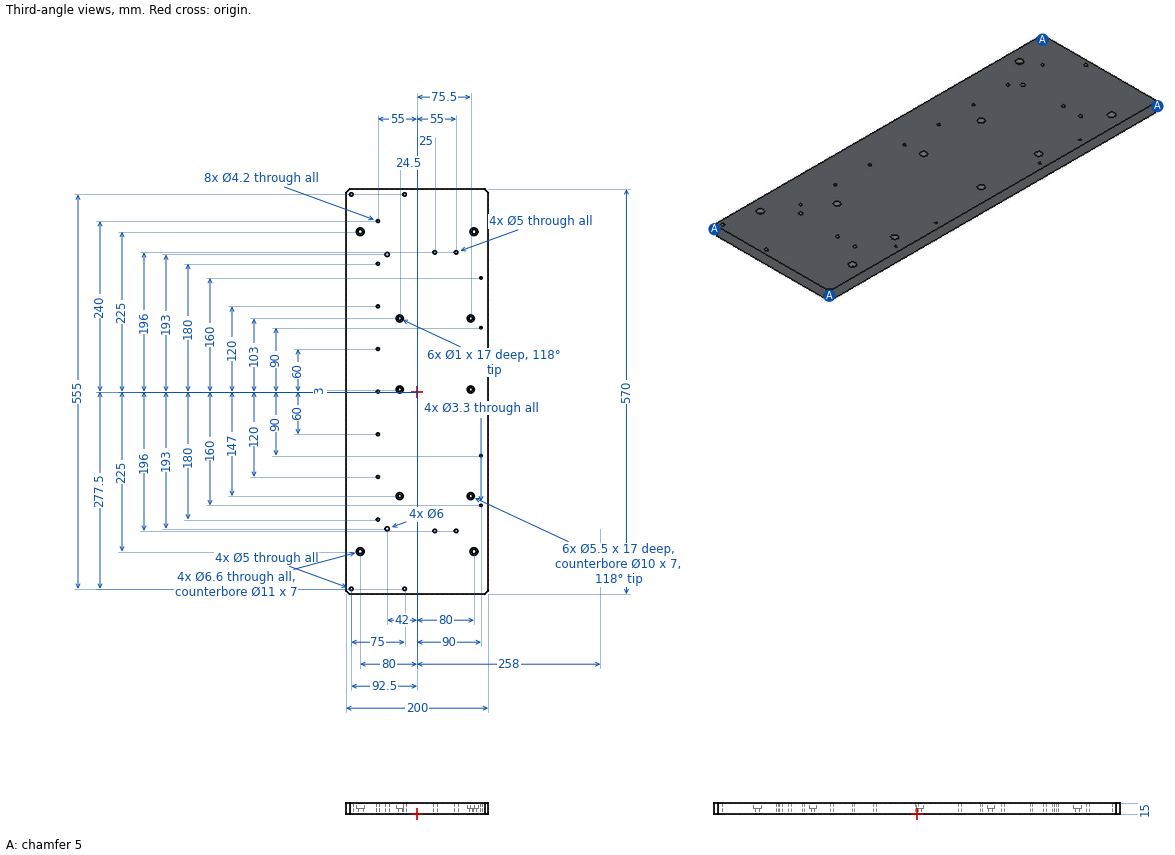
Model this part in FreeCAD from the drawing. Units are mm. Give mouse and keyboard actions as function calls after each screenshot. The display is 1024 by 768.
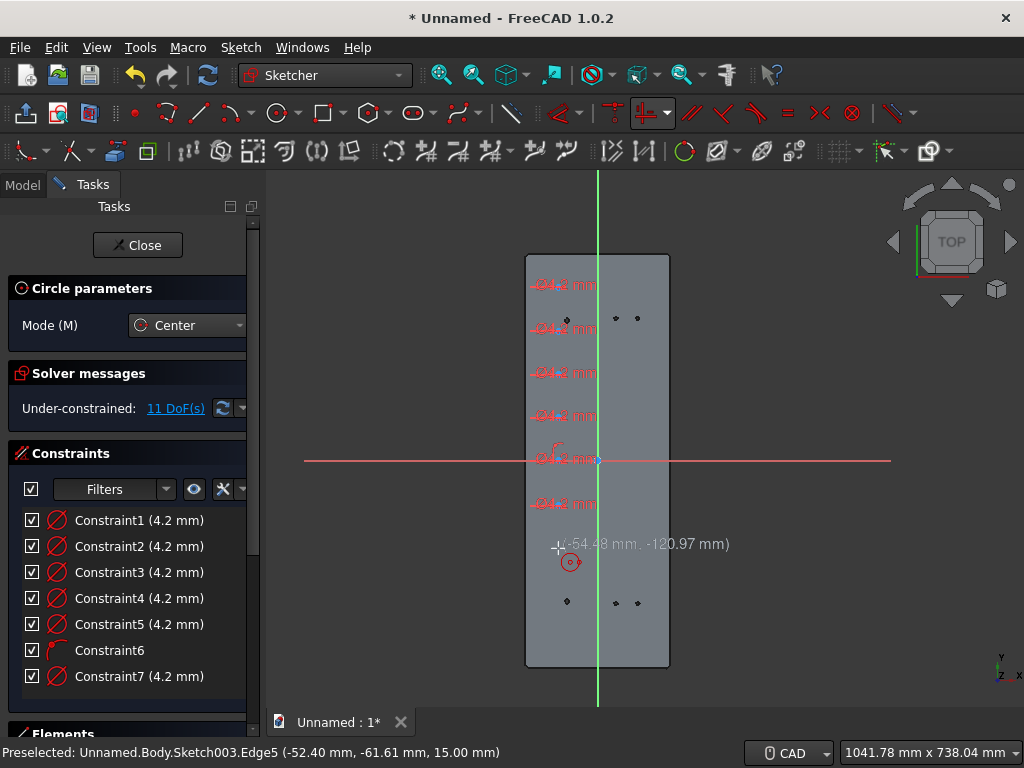
click(558, 548)
move(559, 547)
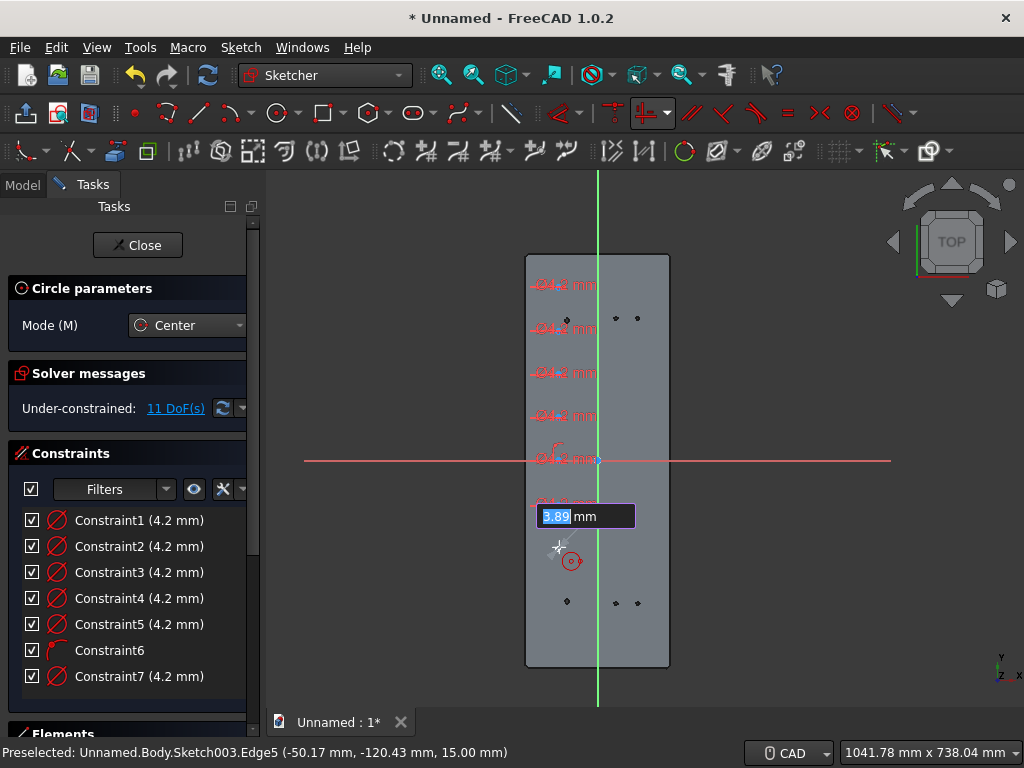
text(4.2)
key(Return)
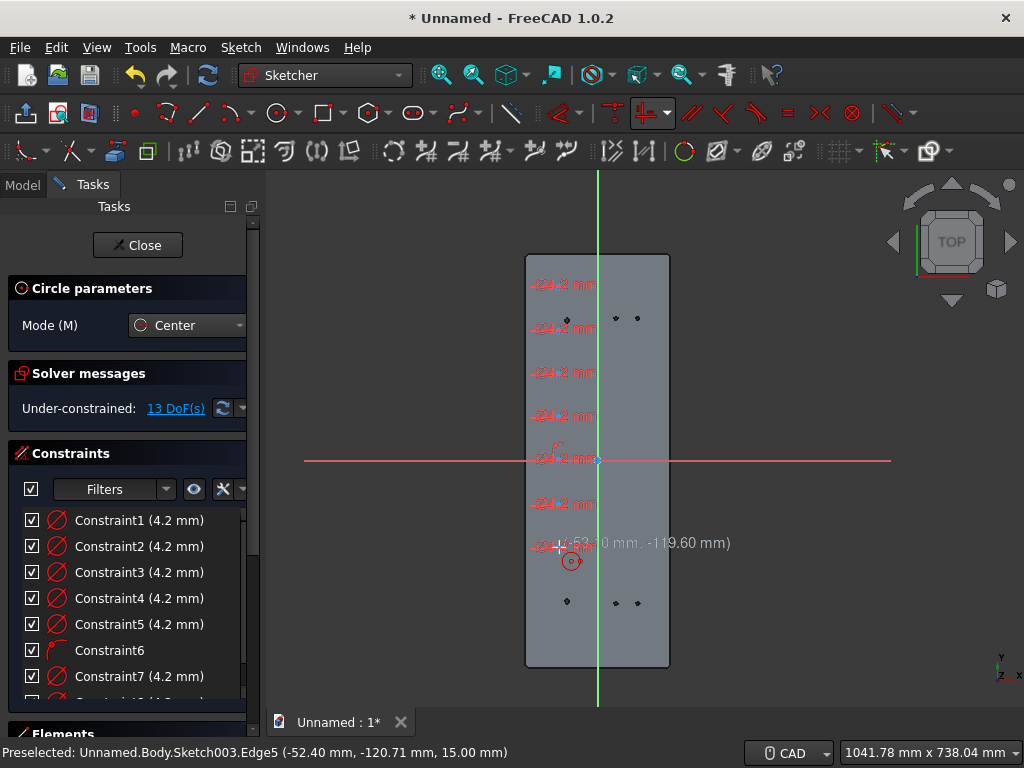
scroll(558, 592, up, 14)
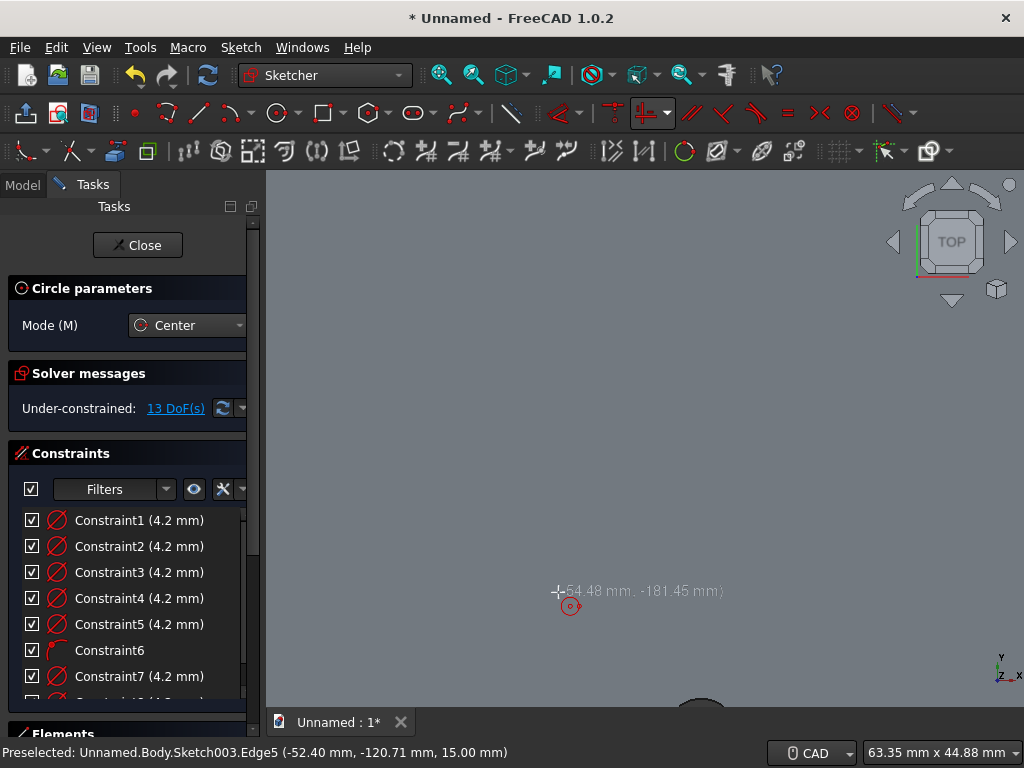
scroll(558, 592, down, 14)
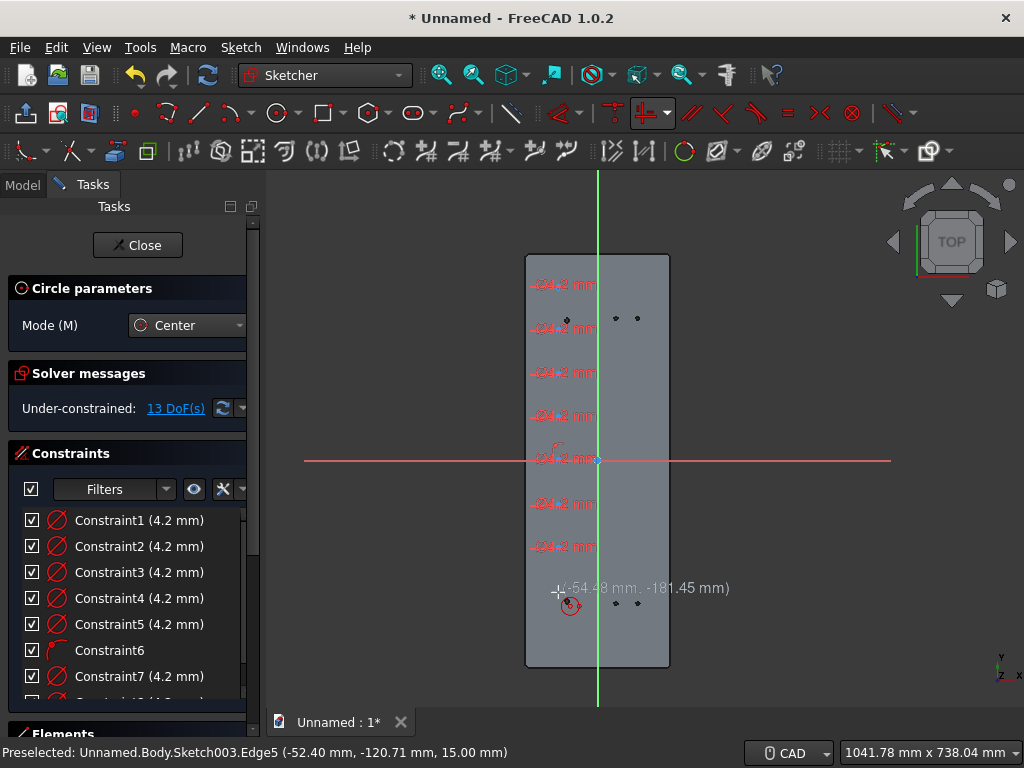
click(558, 592)
move(559, 591)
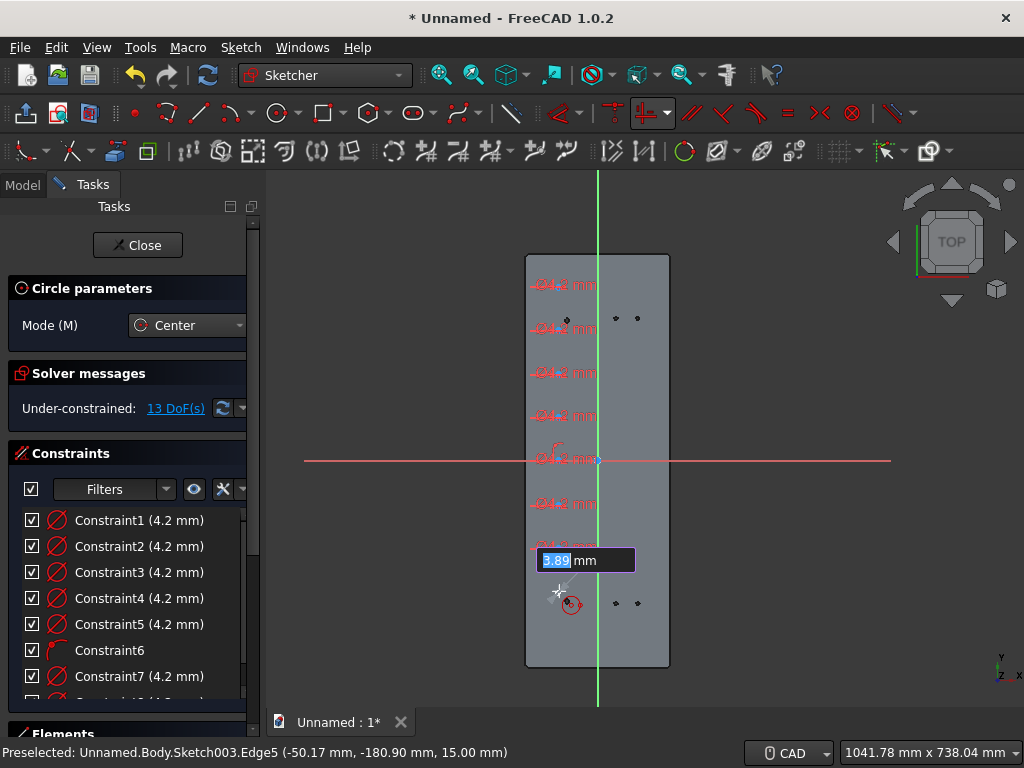
text(4.2)
key(Return)
key(Escape)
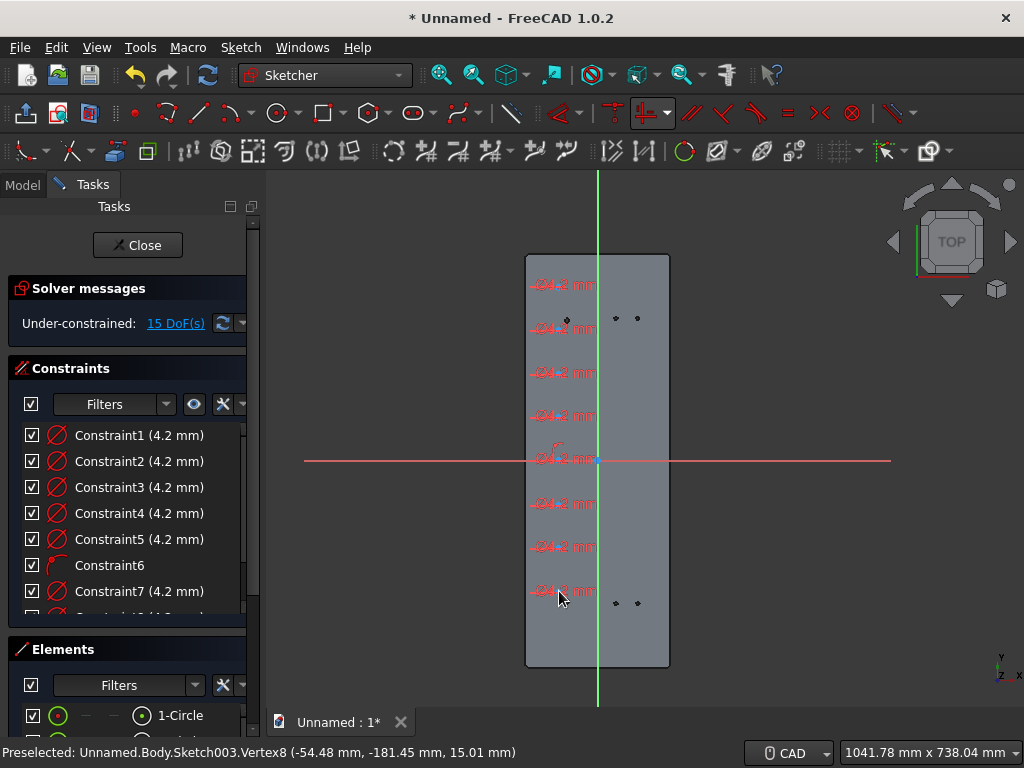
click(558, 287)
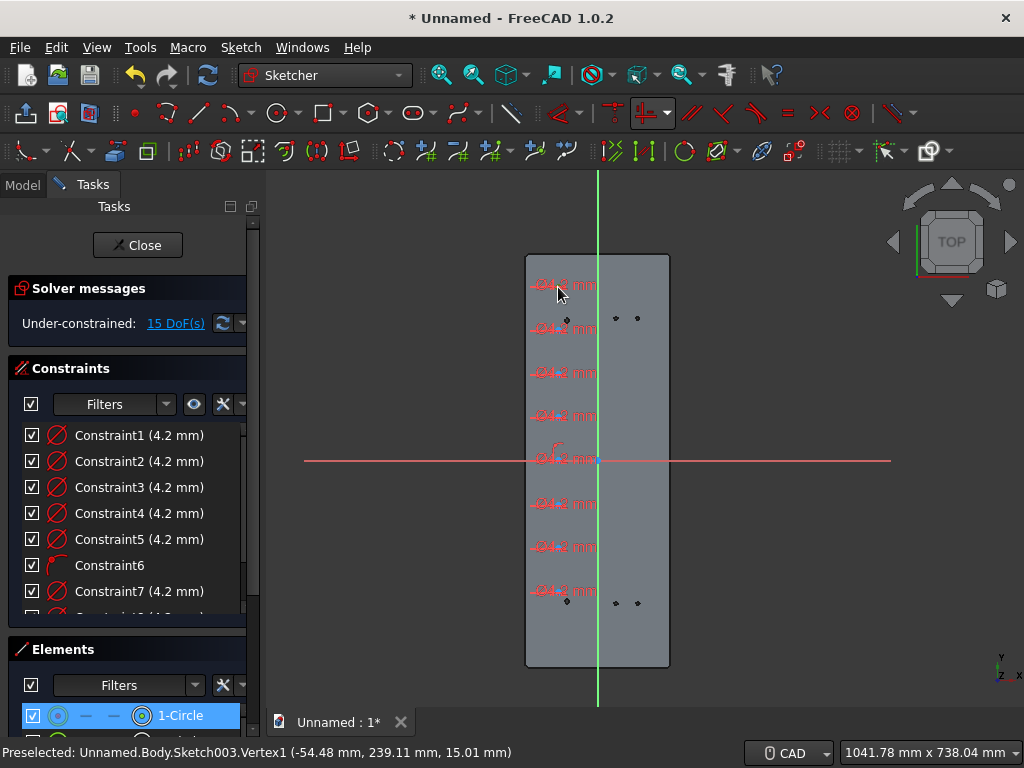
click(558, 331)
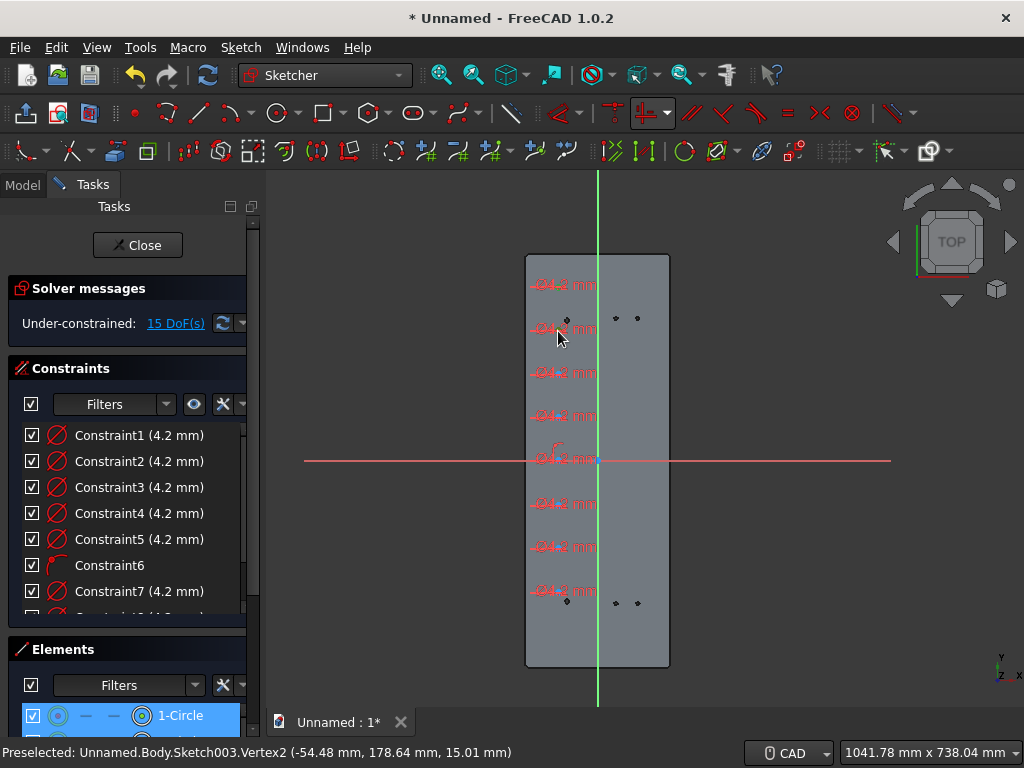
key(v)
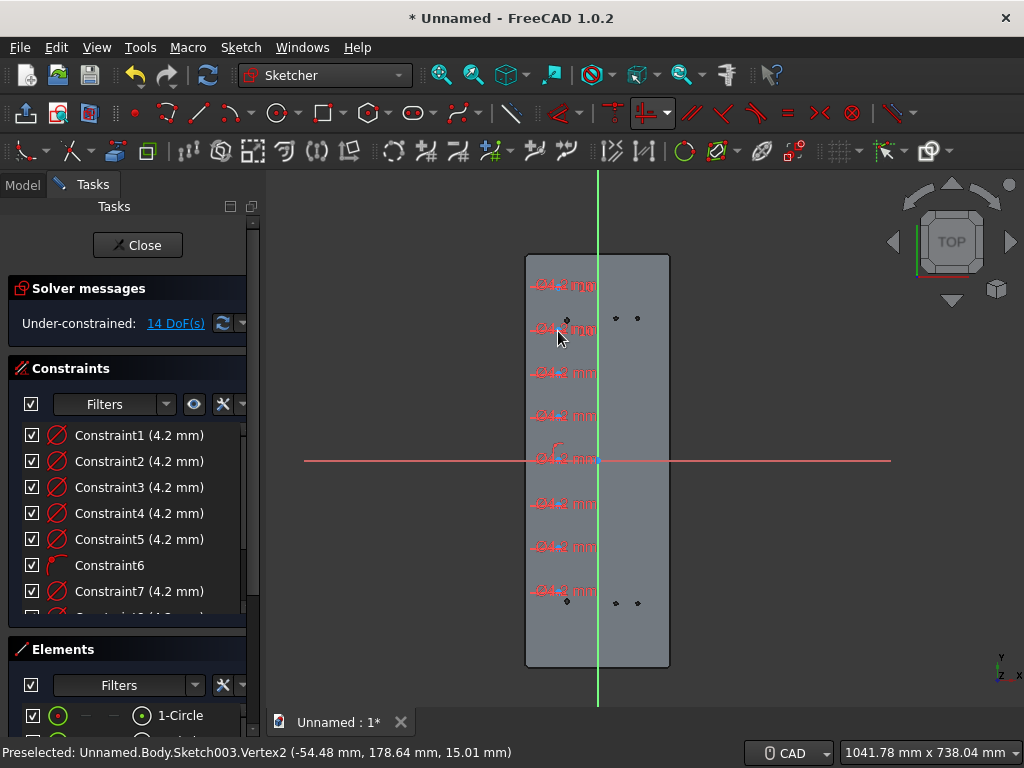
click(558, 331)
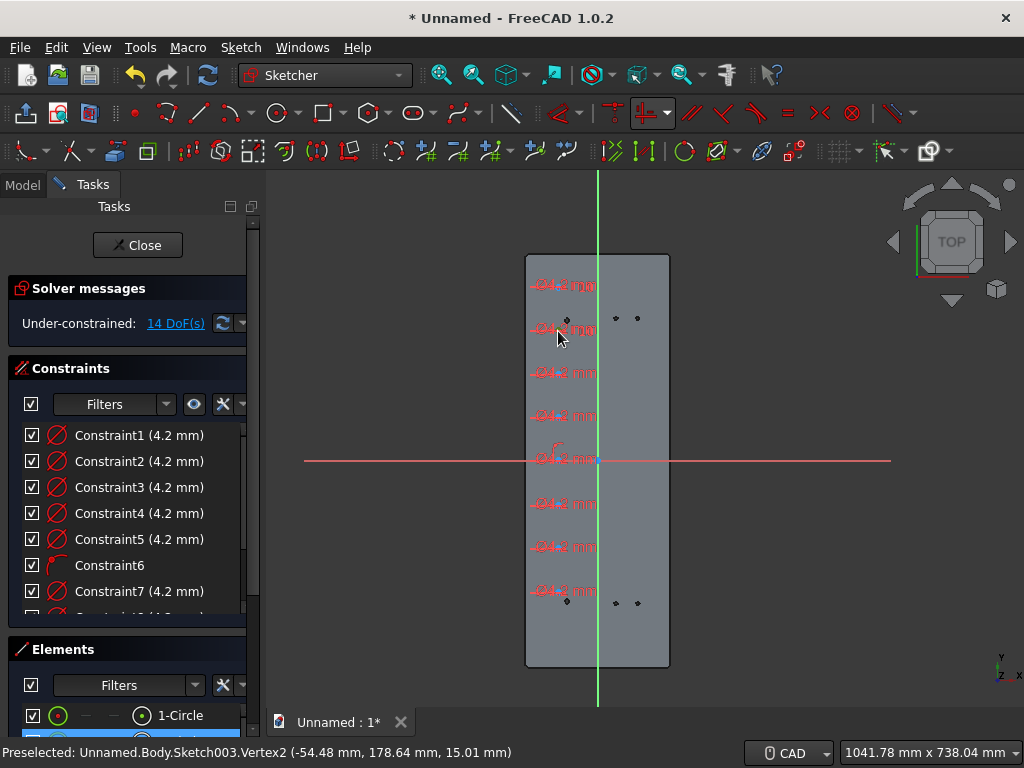
click(558, 375)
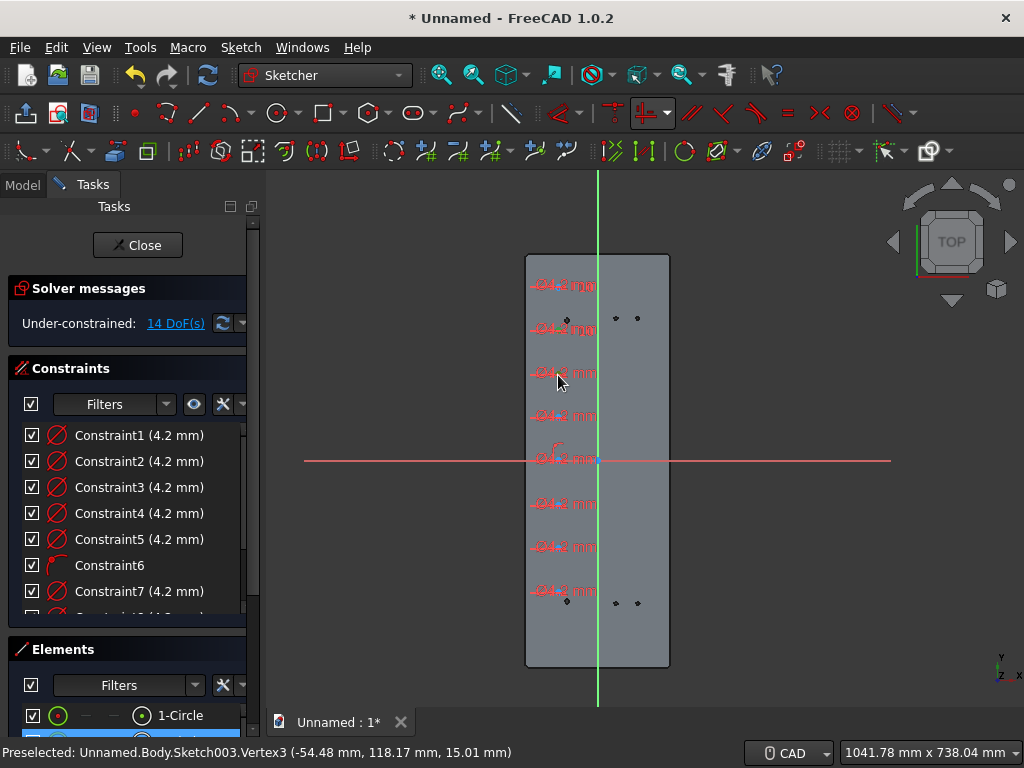
click(670, 114)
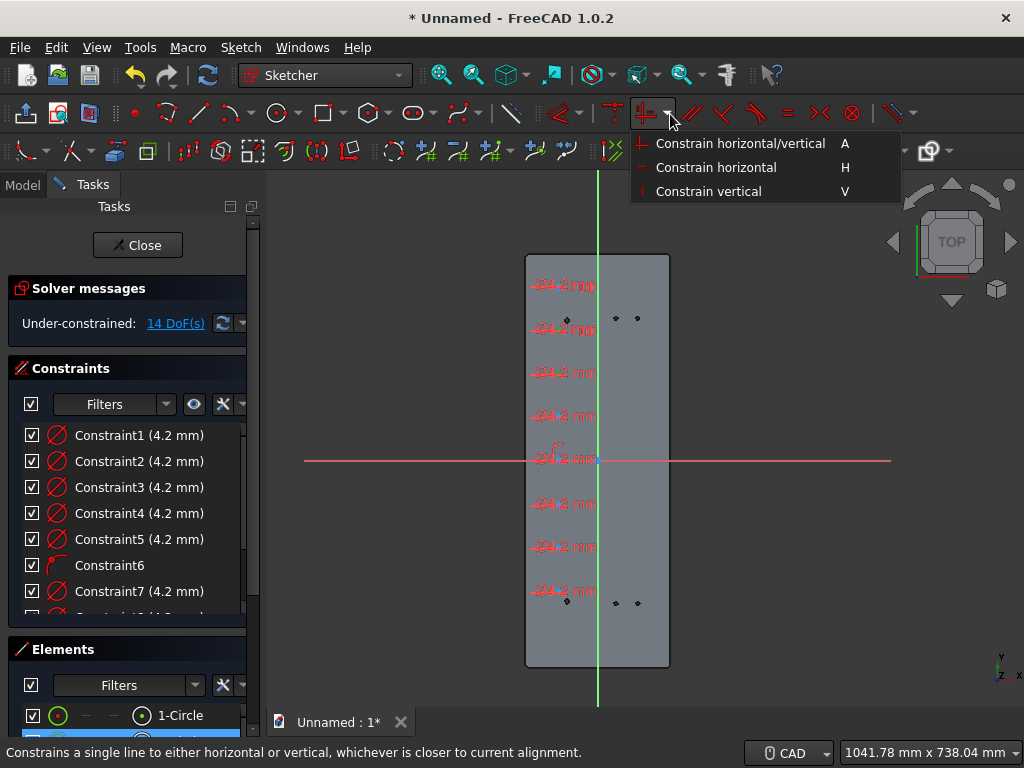
click(766, 191)